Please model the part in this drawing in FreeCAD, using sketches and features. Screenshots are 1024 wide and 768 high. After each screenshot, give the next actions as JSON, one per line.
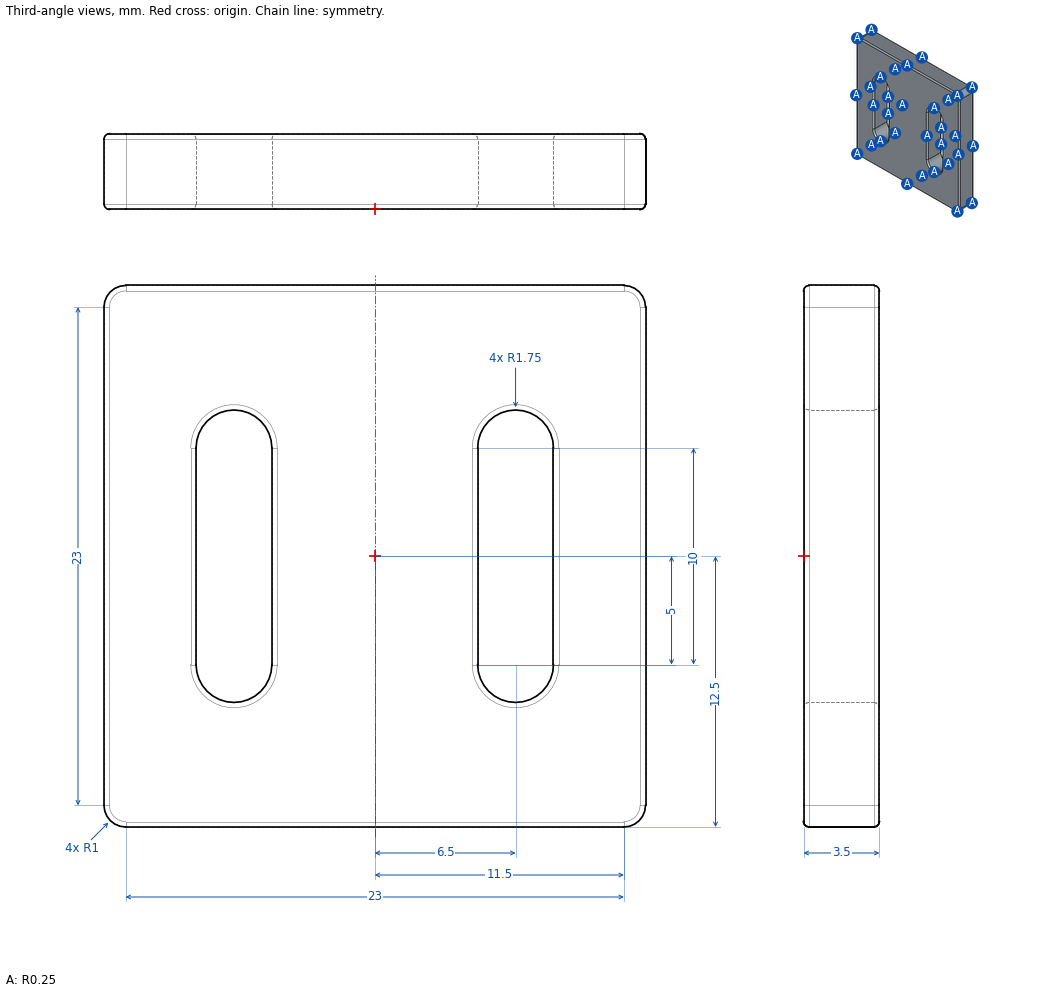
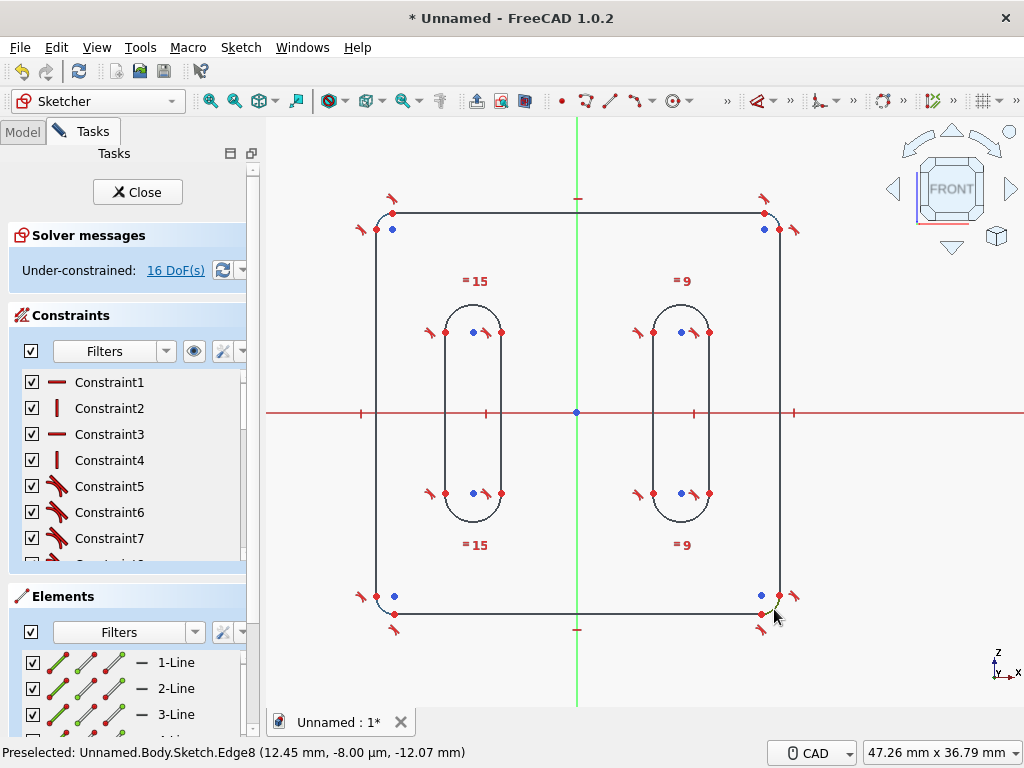
{"action": "key", "text": "e"}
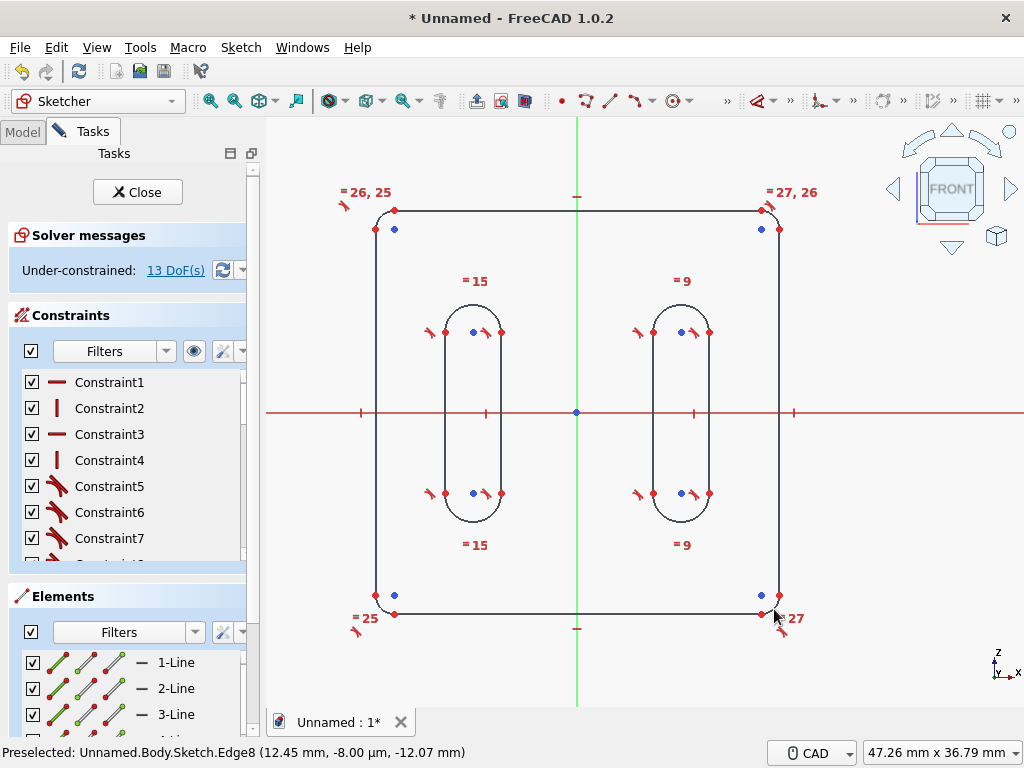
{"action": "left_click", "coordinate": [665, 517]}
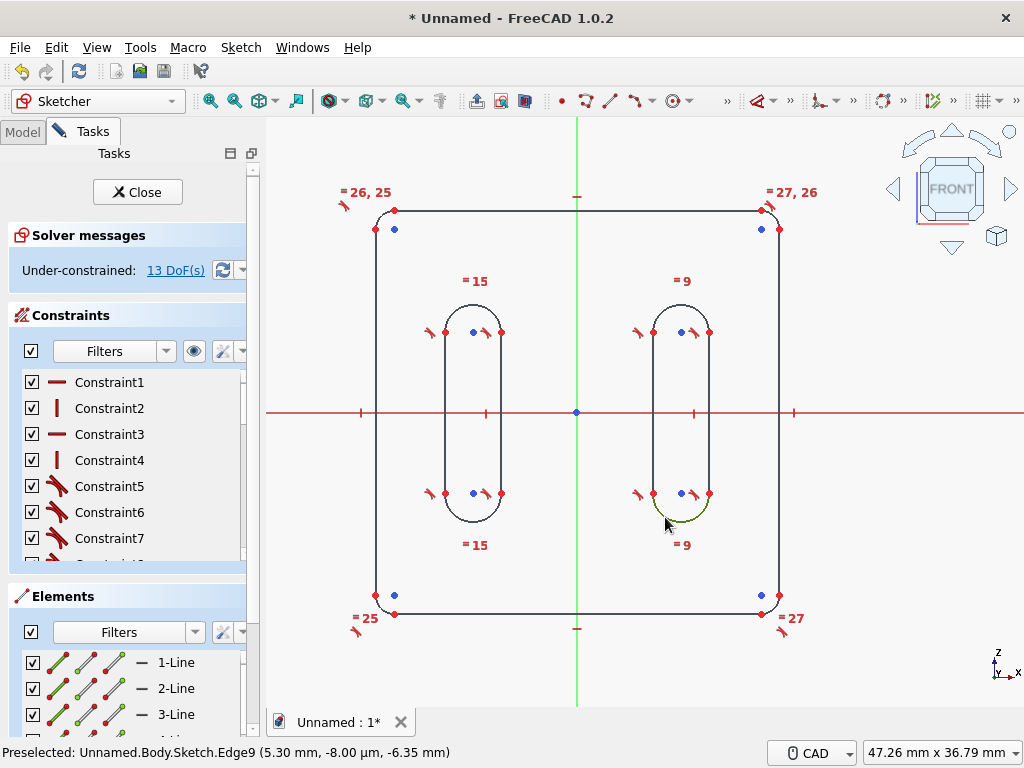
{"action": "left_click", "coordinate": [457, 517]}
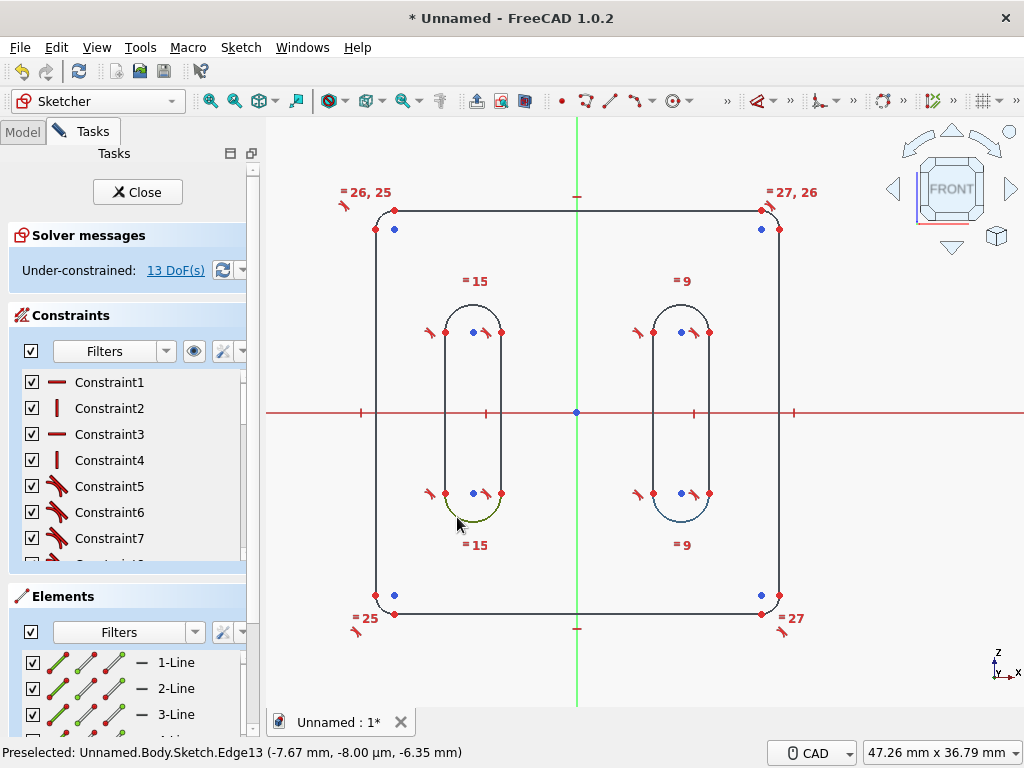
{"action": "key", "text": "e"}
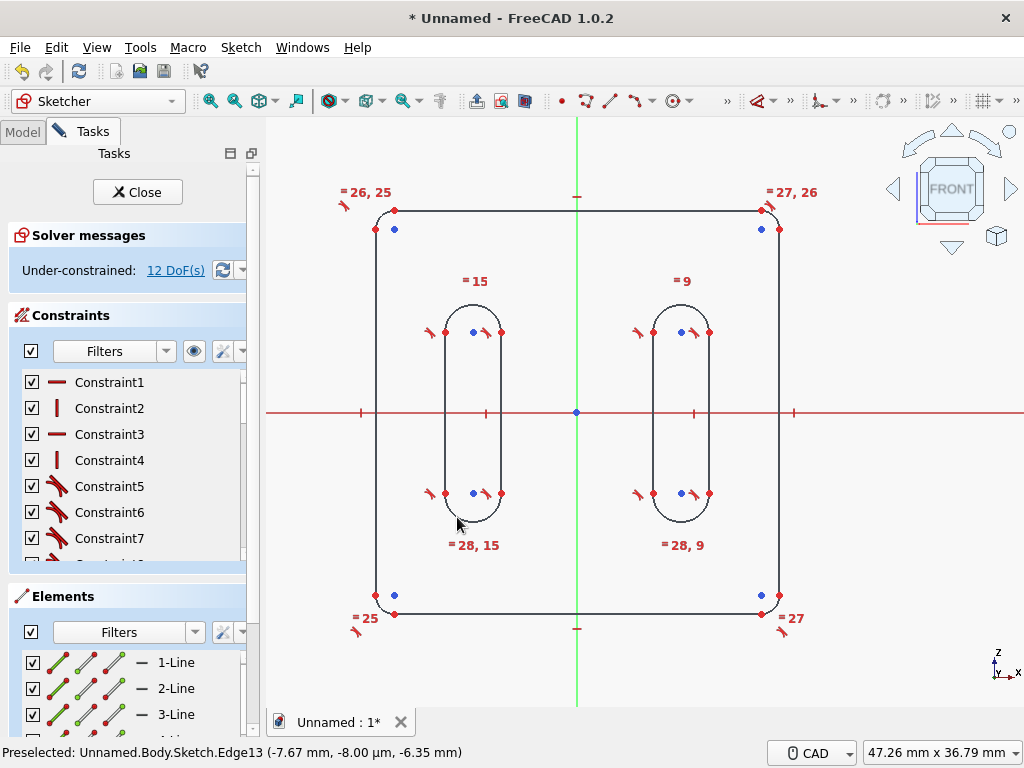
{"action": "left_click", "coordinate": [681, 494]}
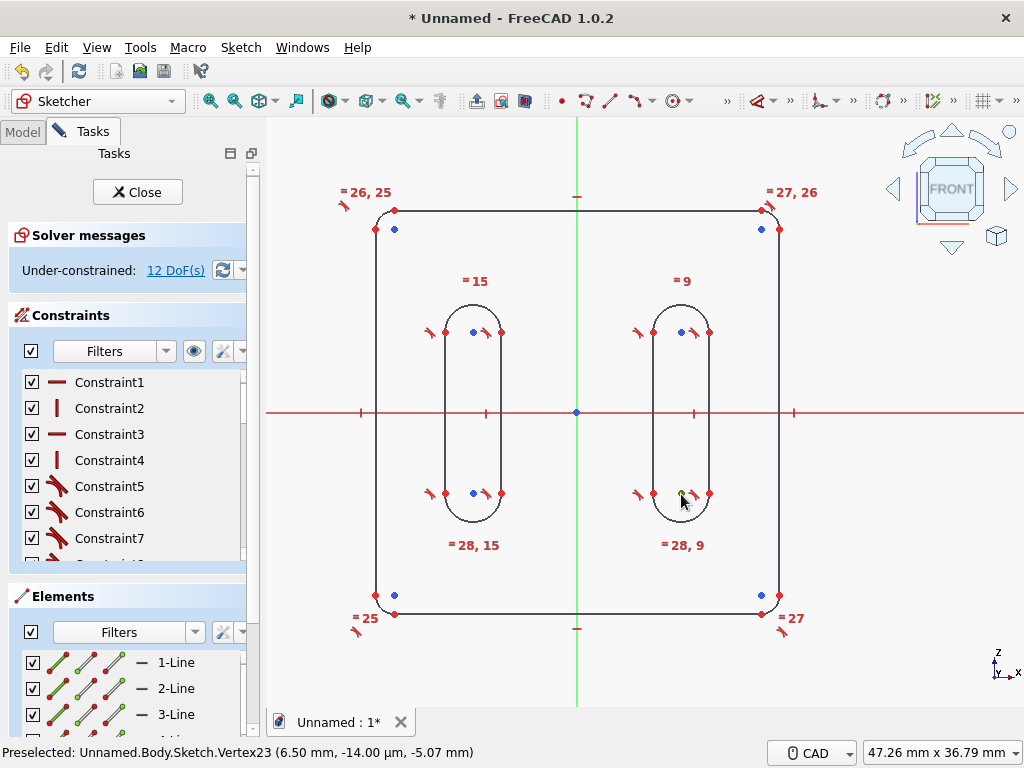
{"action": "left_click", "coordinate": [473, 494]}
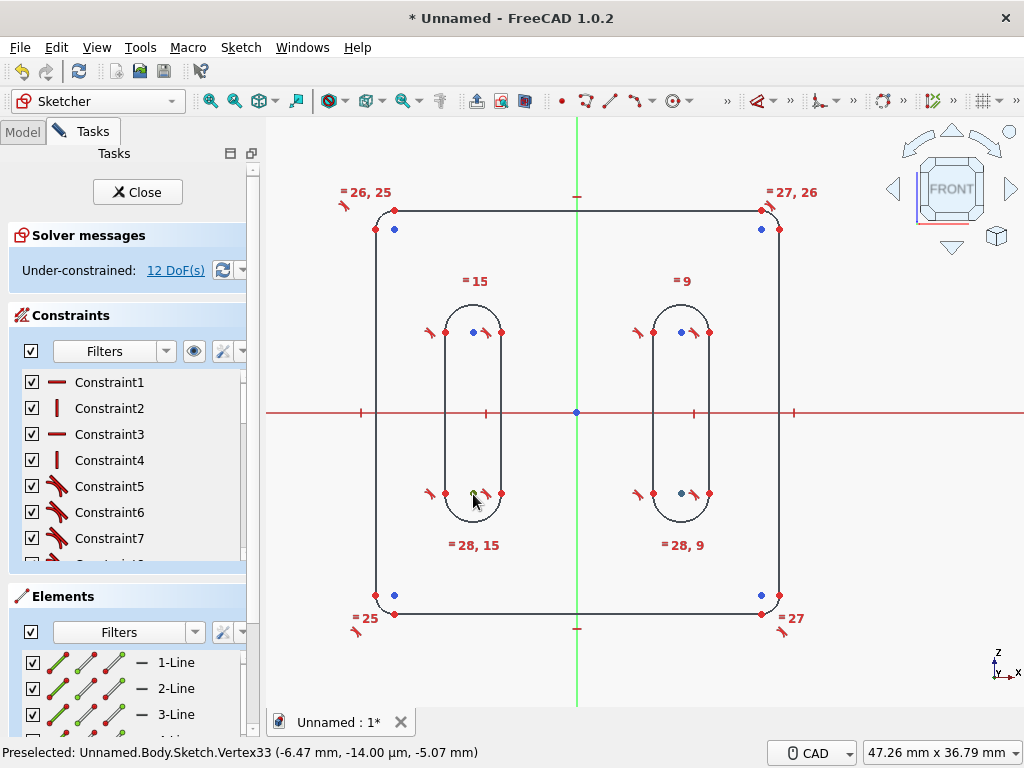
{"action": "left_click", "coordinate": [577, 565]}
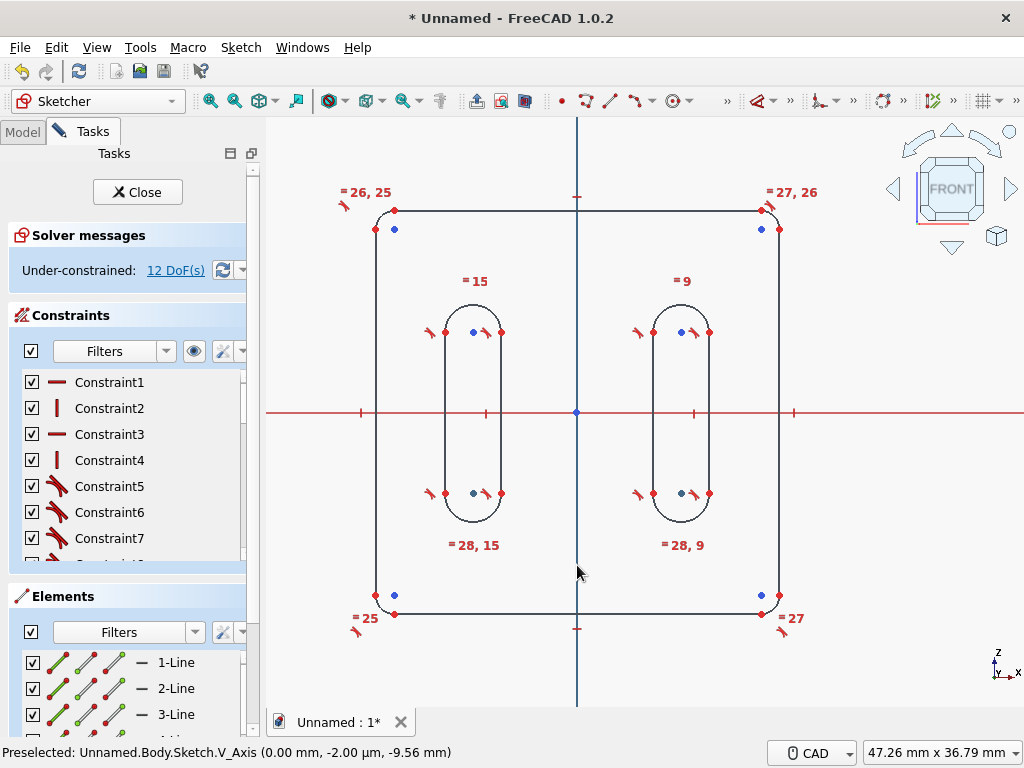
{"action": "key", "text": "s"}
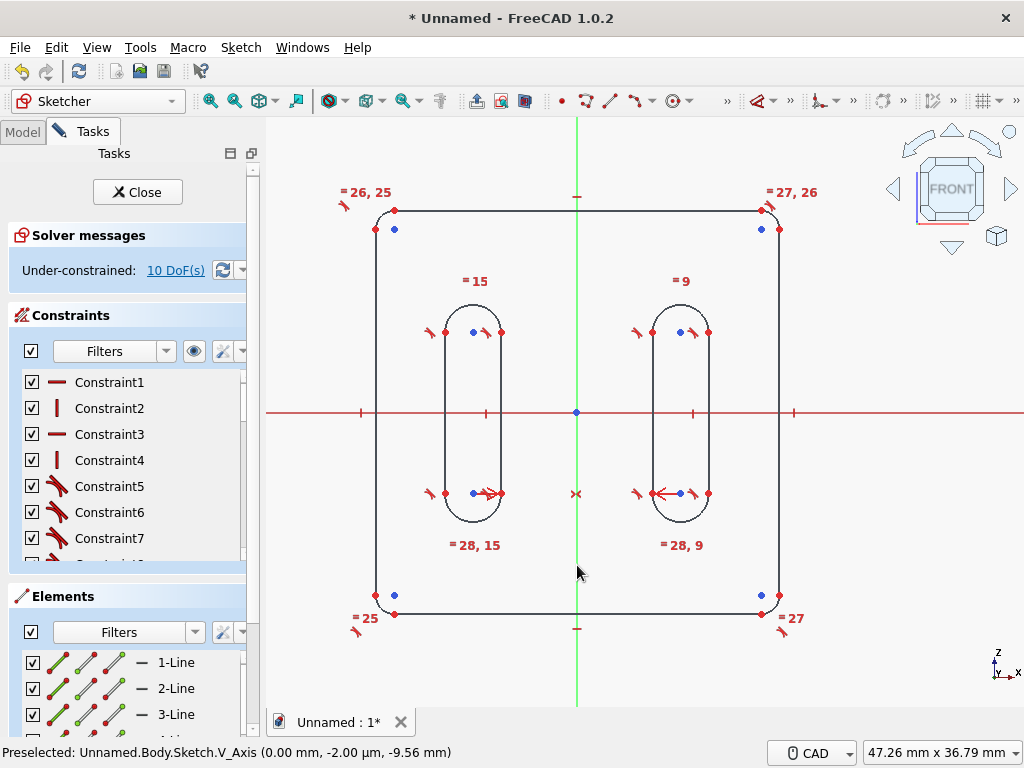
{"action": "scroll", "coordinate": [381, 609], "scroll_direction": "up", "scroll_amount": 5}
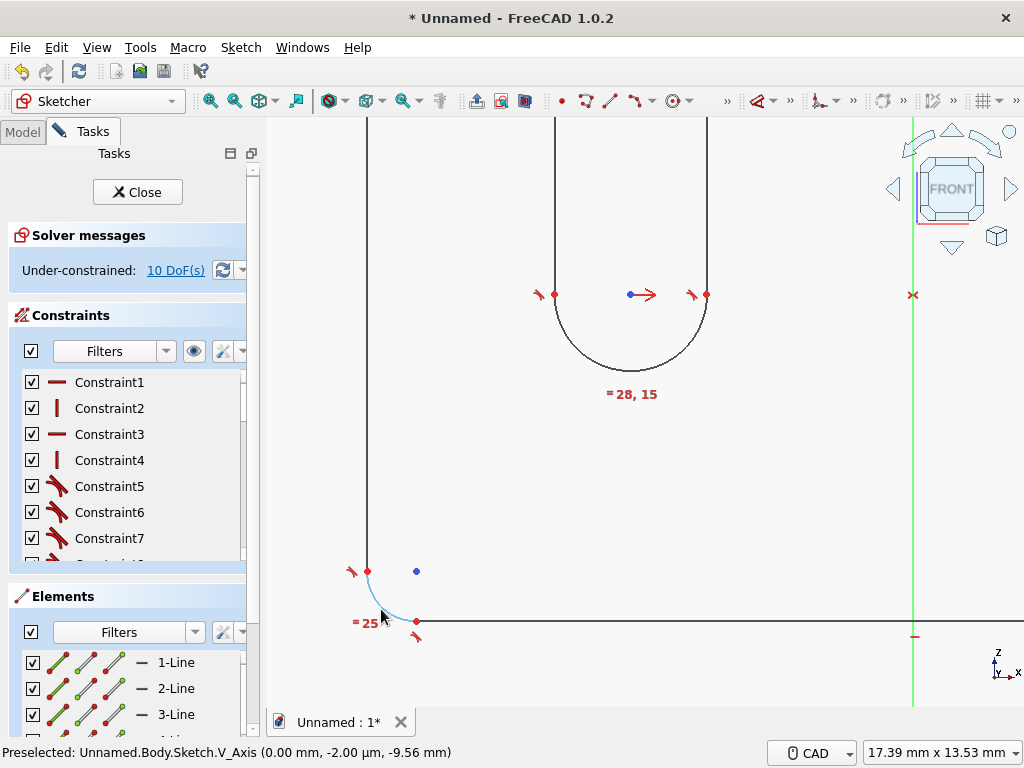
{"action": "left_click", "coordinate": [382, 607]}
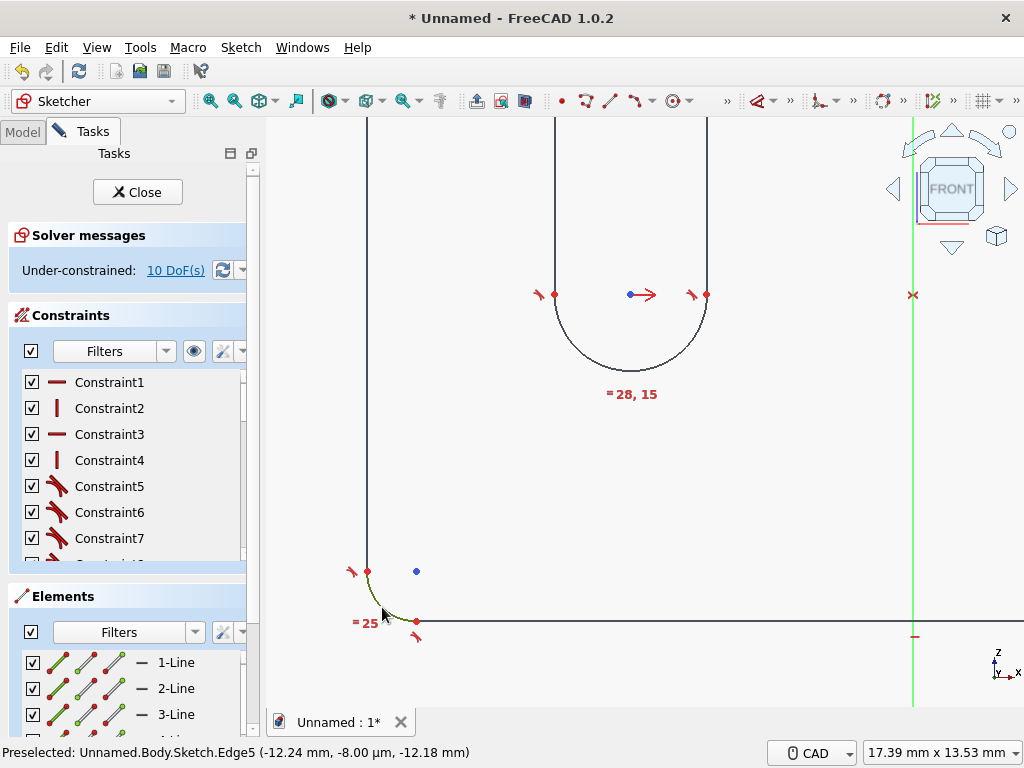
{"action": "left_click", "coordinate": [776, 102]}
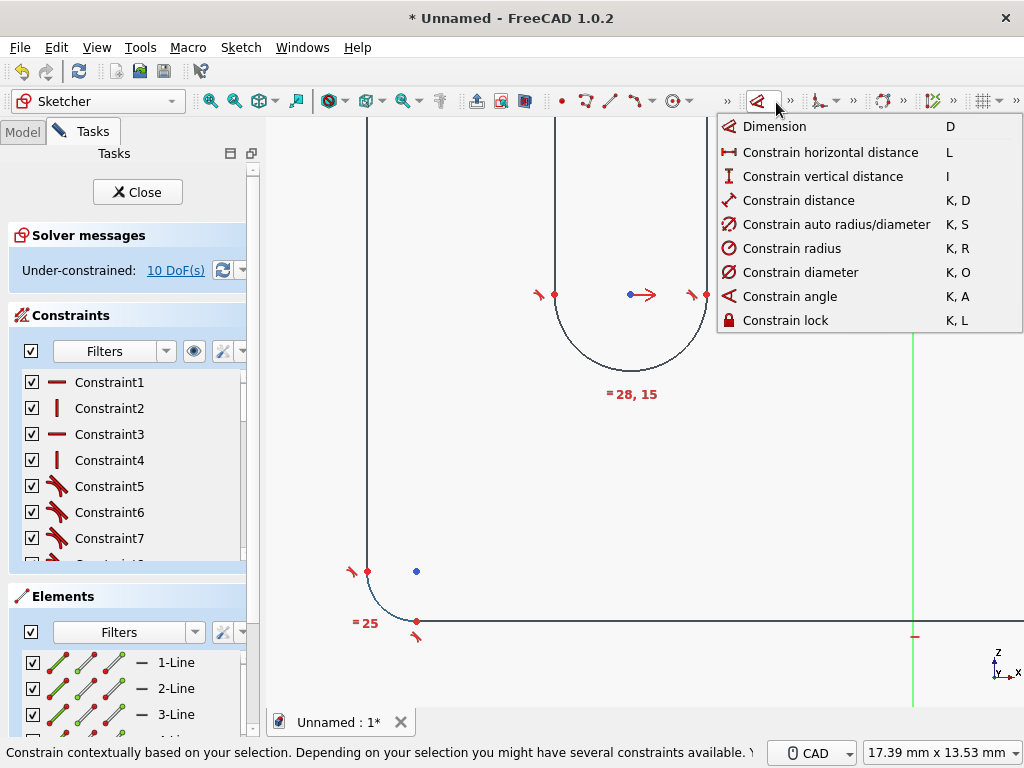
{"action": "left_click", "coordinate": [870, 248]}